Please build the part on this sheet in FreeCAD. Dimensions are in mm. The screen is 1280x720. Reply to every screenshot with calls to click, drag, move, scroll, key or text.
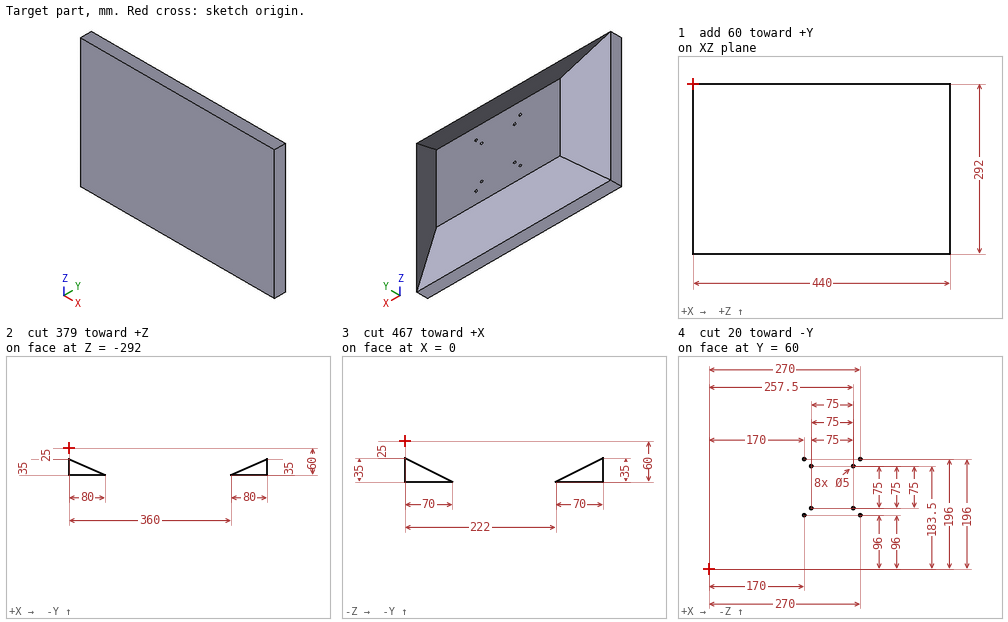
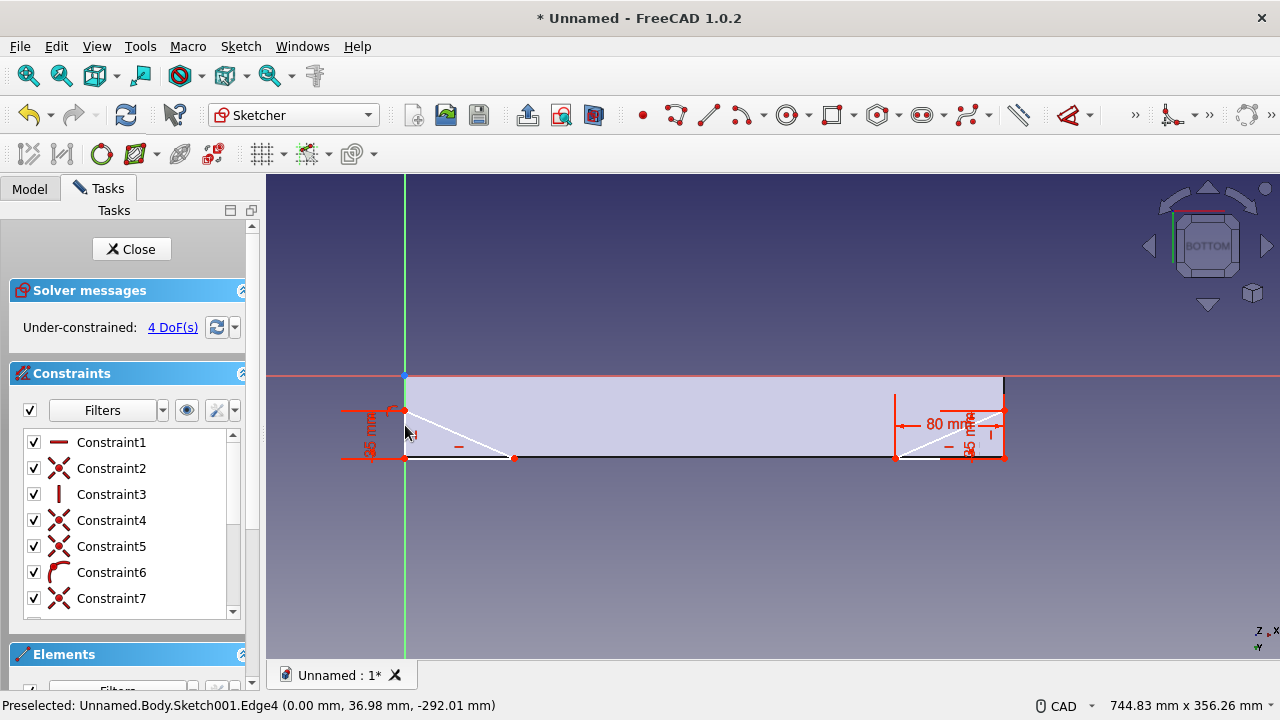
click(438, 459)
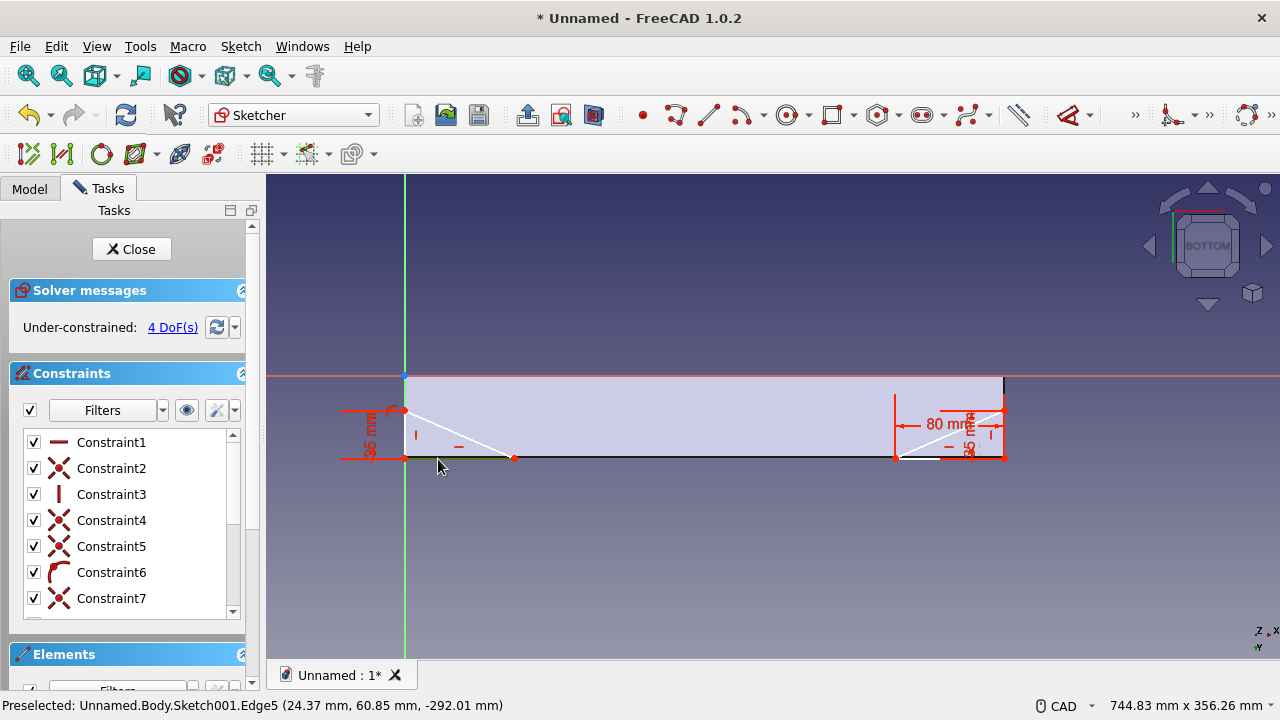
click(1090, 116)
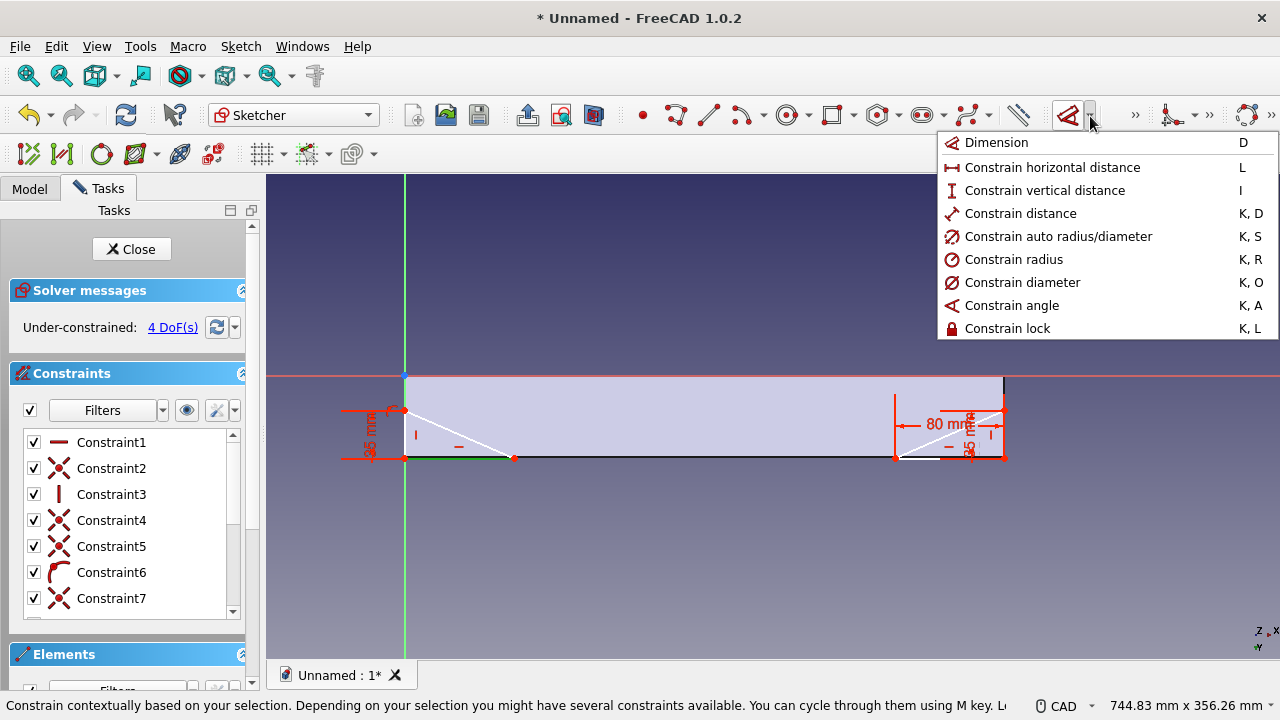
click(1108, 168)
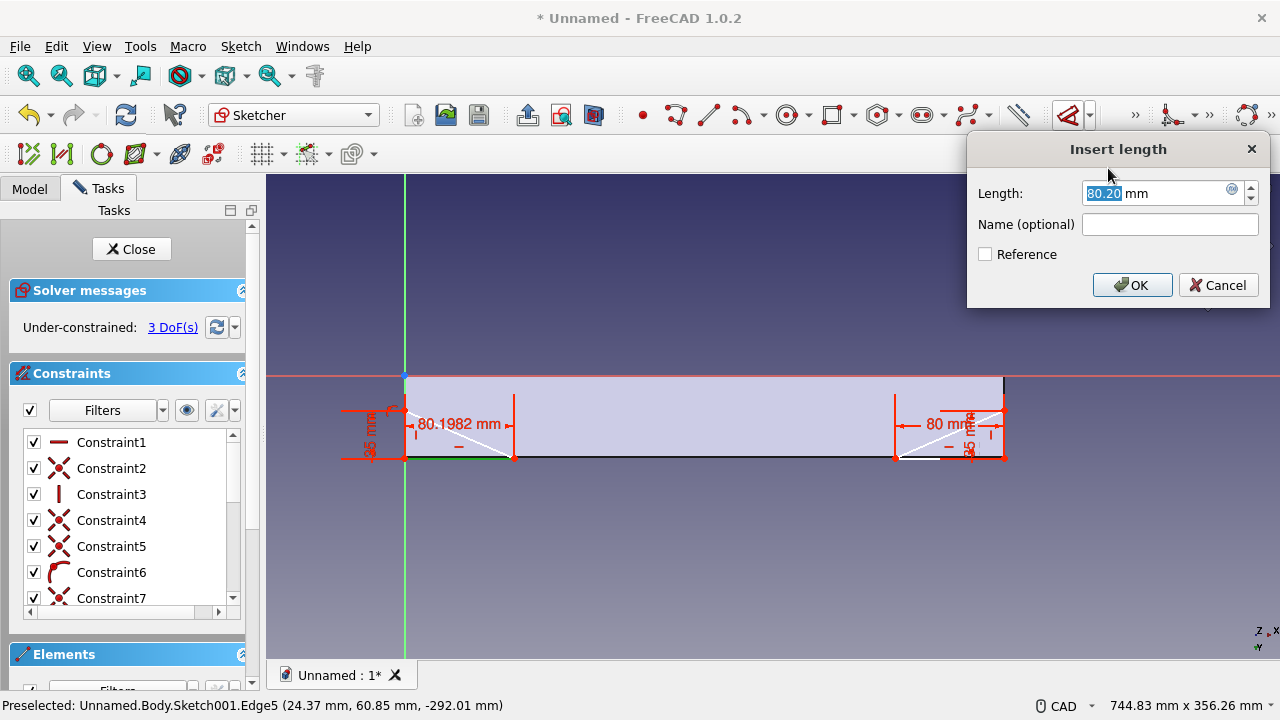
text(80)
key(Return)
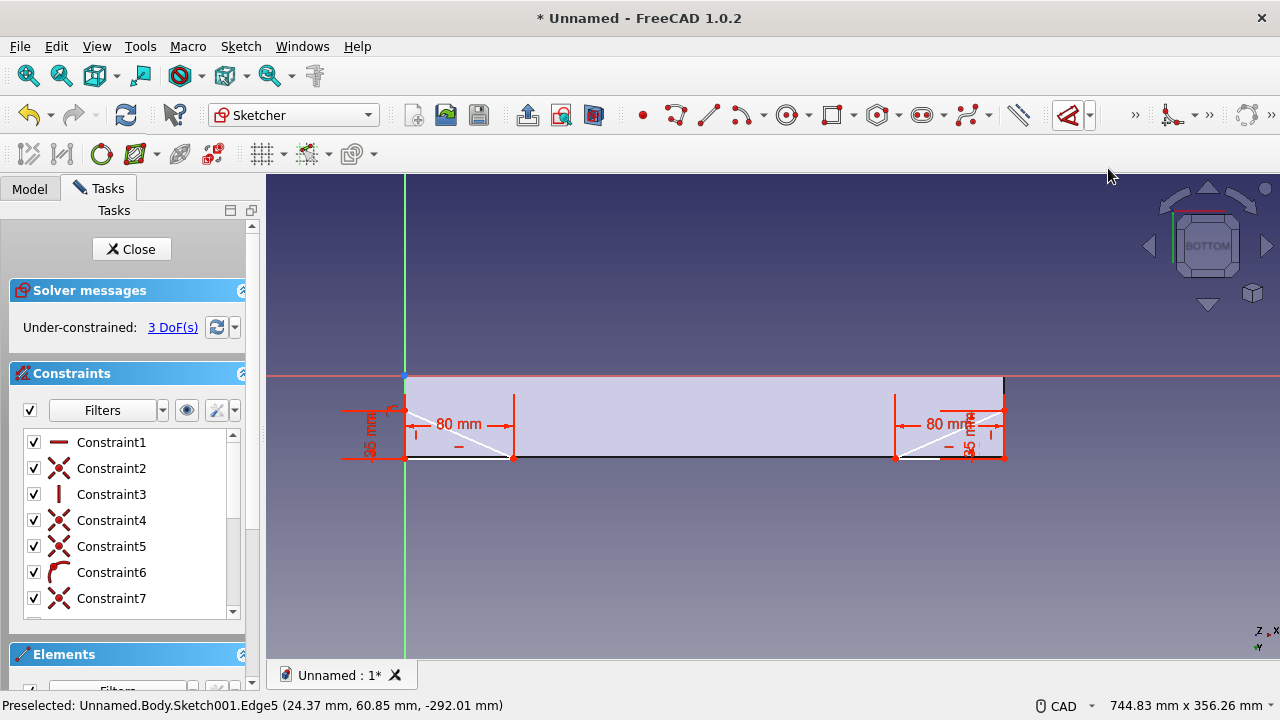
click(895, 459)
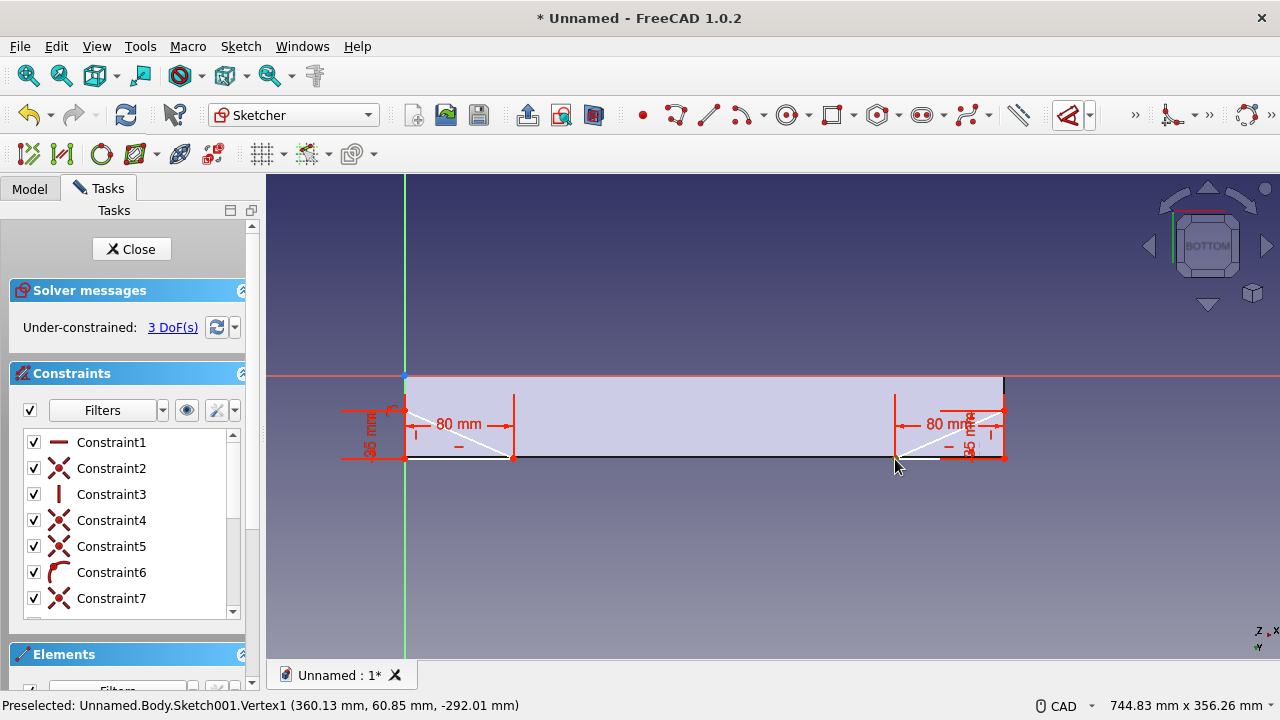
key(i)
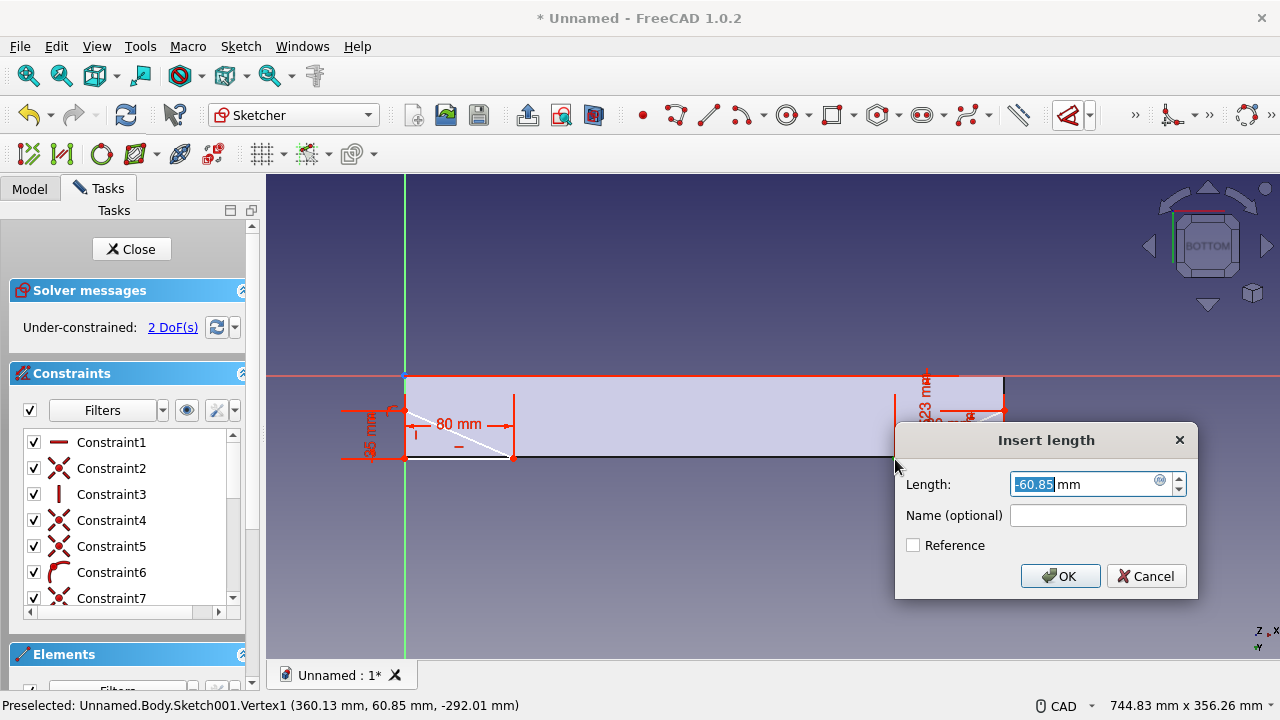
text(-60)
key(Return)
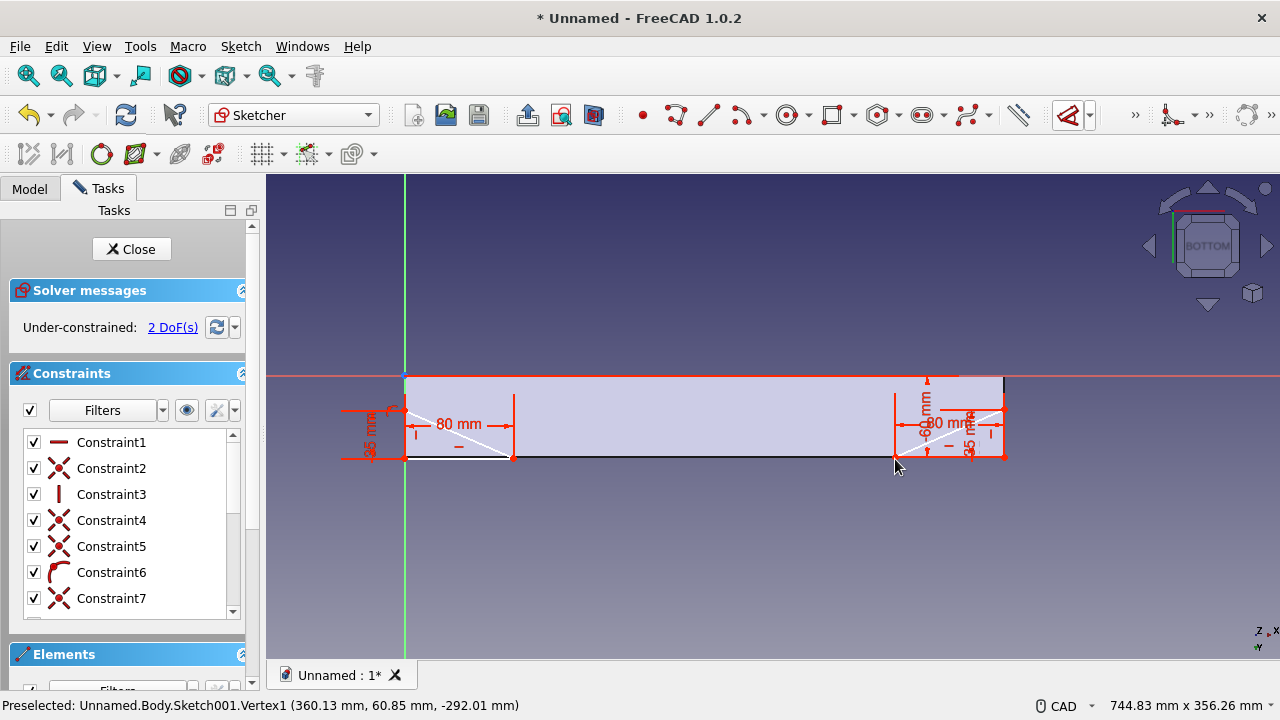
click(405, 411)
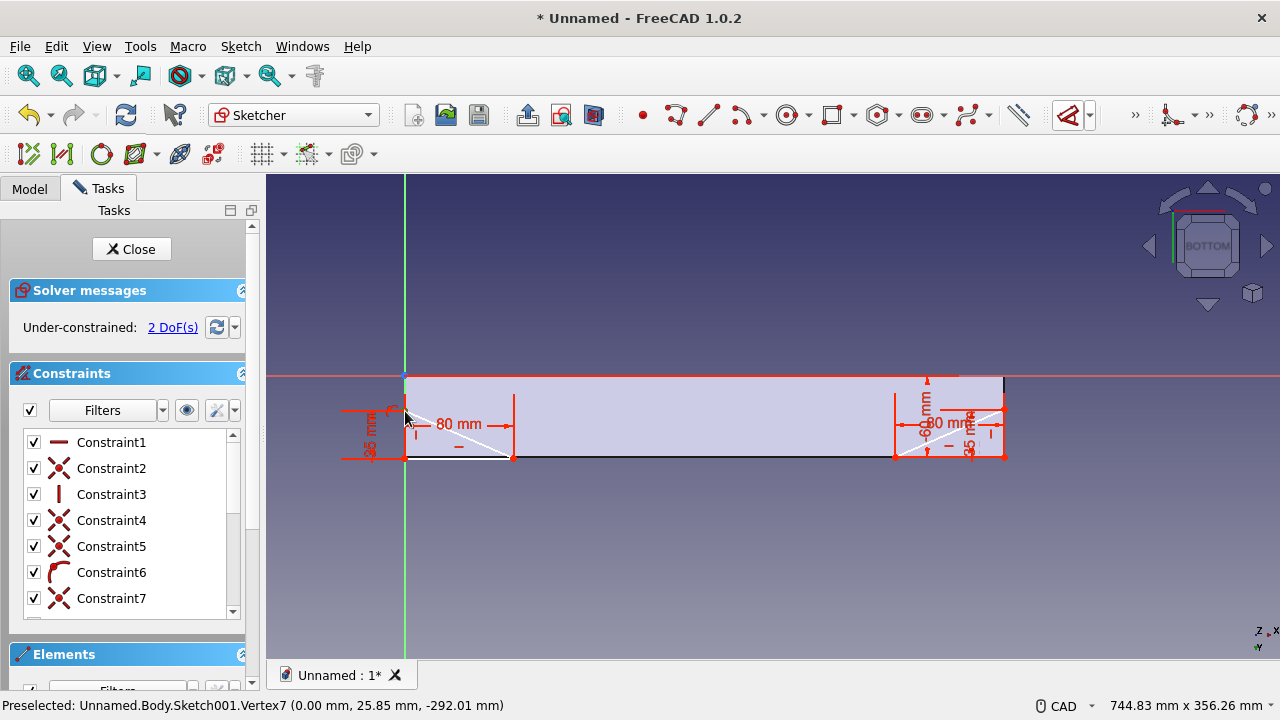
key(i)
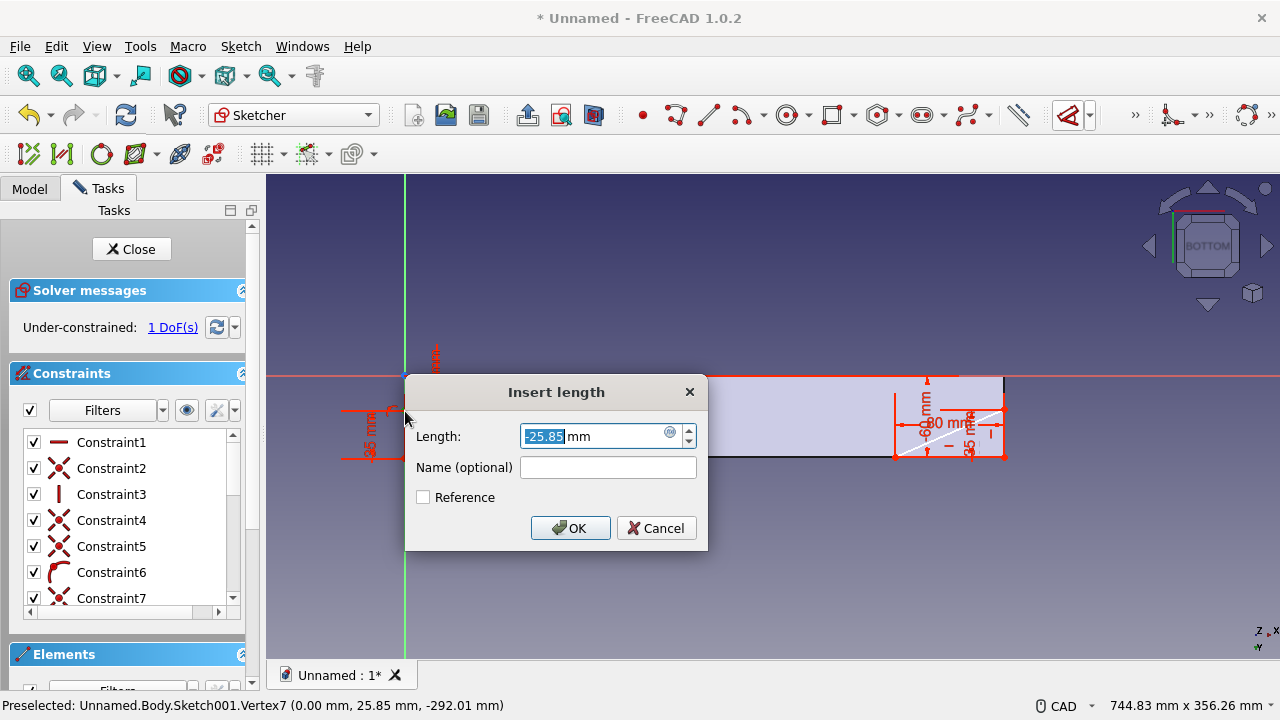
text(-25)
key(Return)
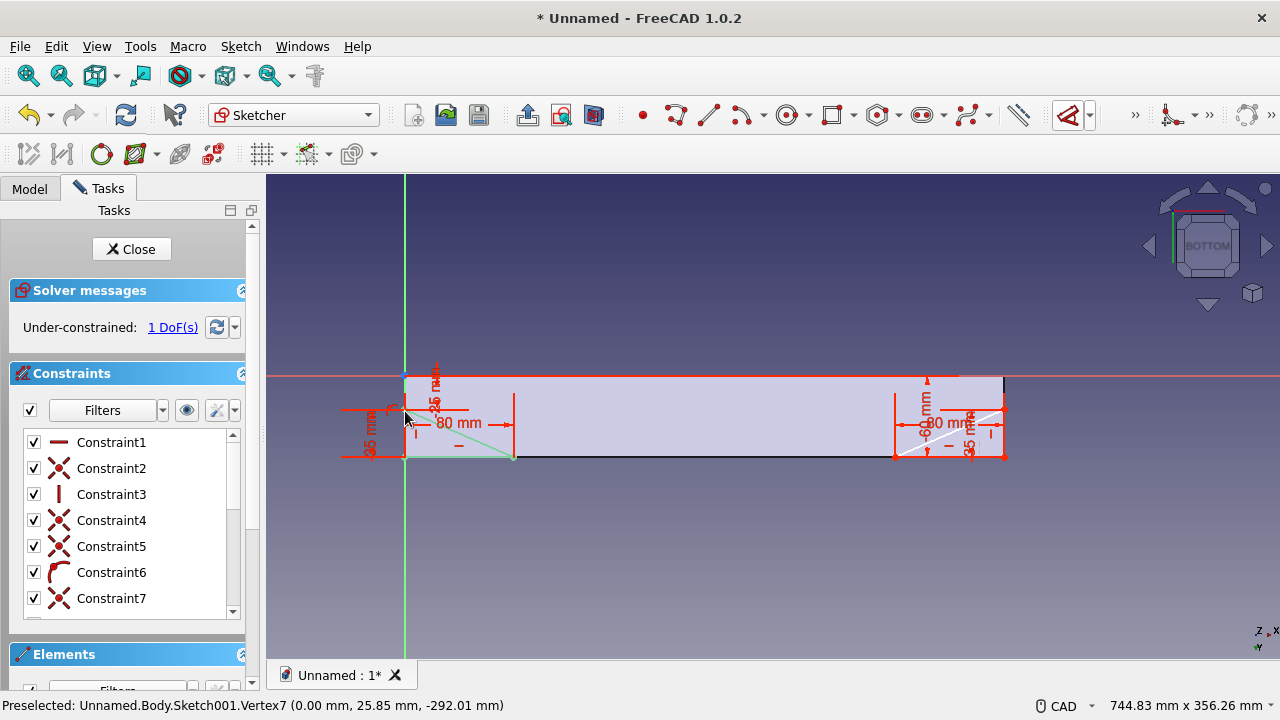
click(895, 457)